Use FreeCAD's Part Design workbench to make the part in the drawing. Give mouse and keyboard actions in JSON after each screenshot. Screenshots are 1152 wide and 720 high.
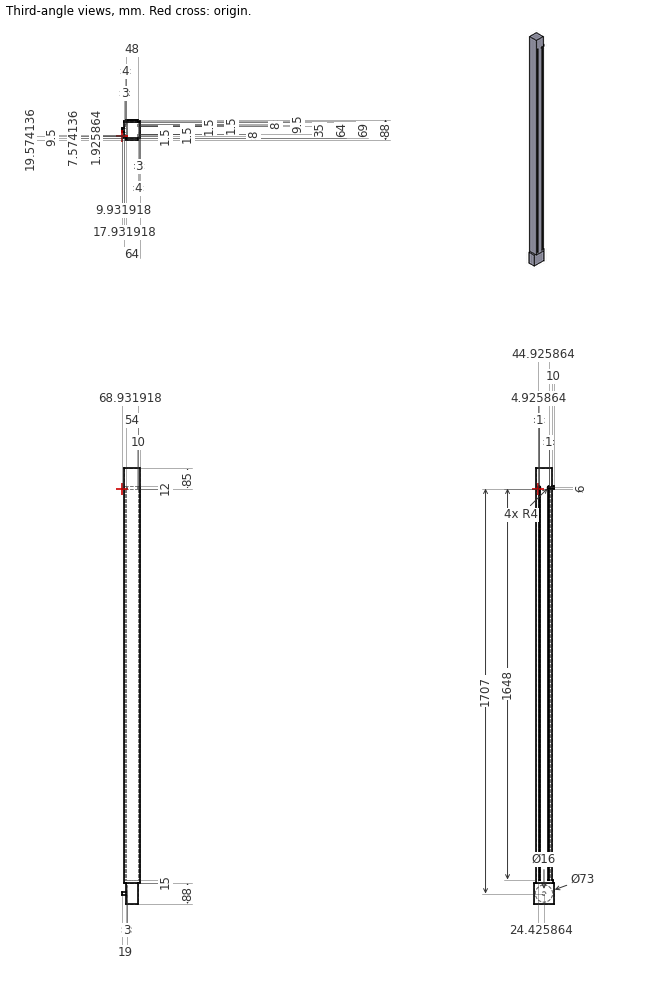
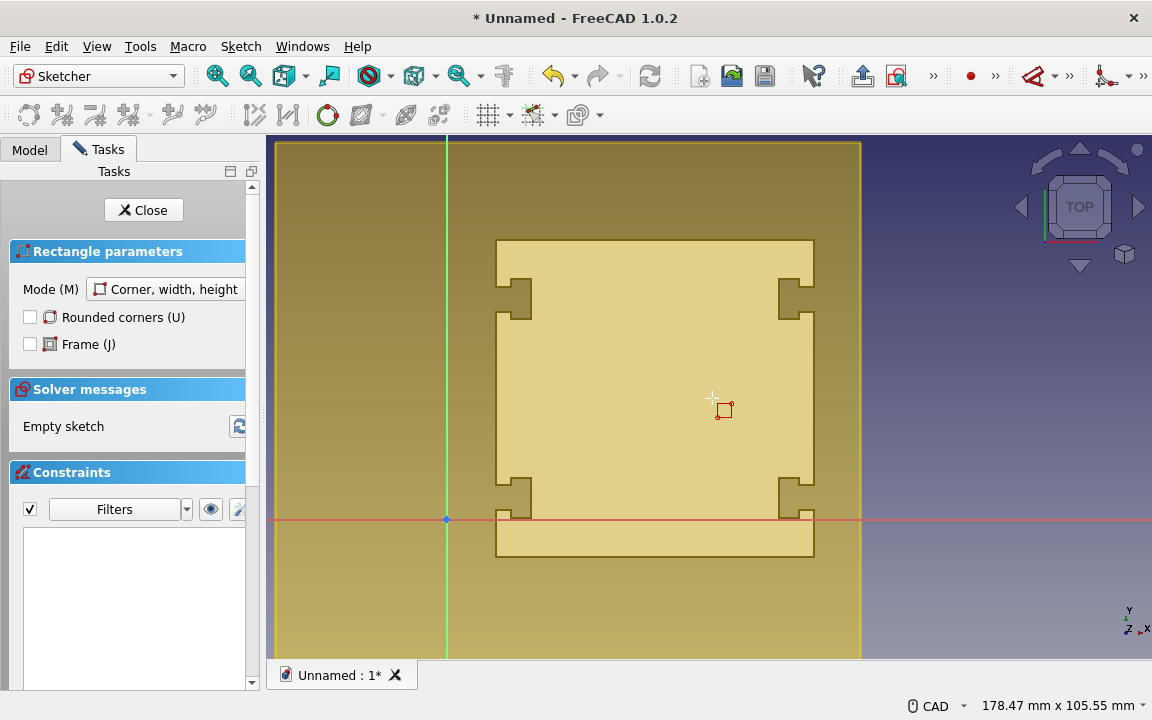
{"action": "left_click", "coordinate": [496, 215]}
{"action": "mouse_move", "coordinate": [814, 557]}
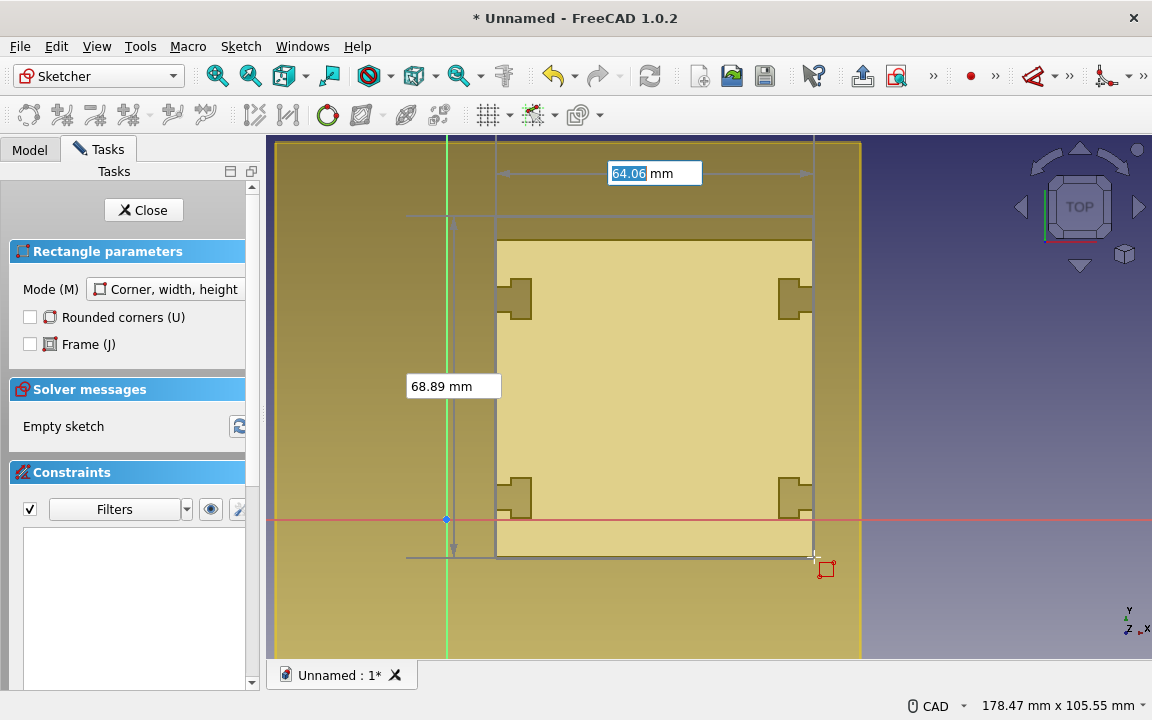
{"action": "type", "text": "64"}
{"action": "key", "text": "Tab"}
{"action": "type", "text": "69"}
{"action": "key", "text": "Return"}
{"action": "key", "text": "Escape"}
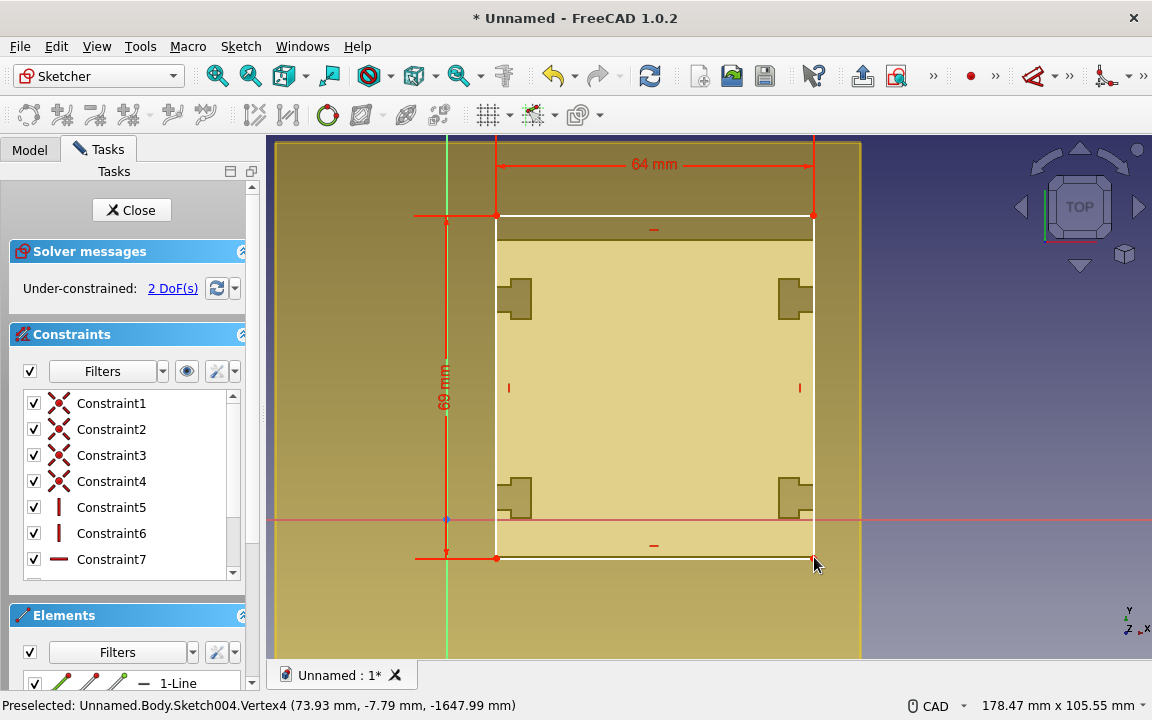
{"action": "left_click", "coordinate": [1032, 76]}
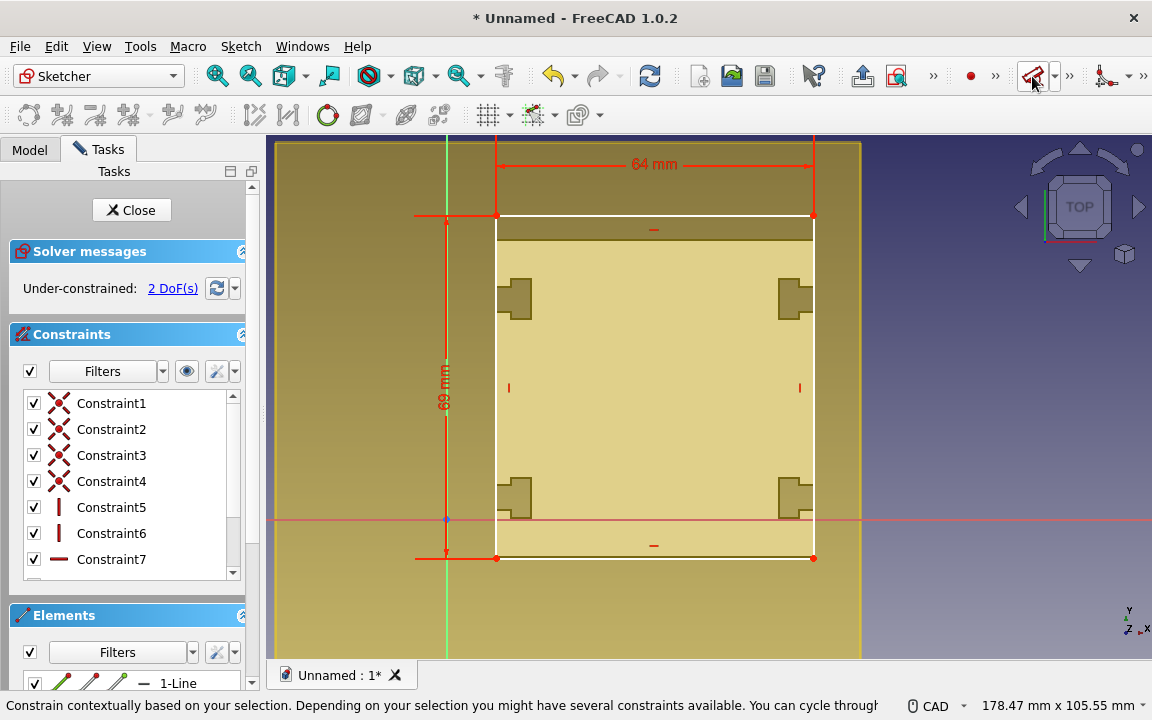
{"action": "left_click", "coordinate": [496, 216]}
{"action": "left_click", "coordinate": [471, 182]}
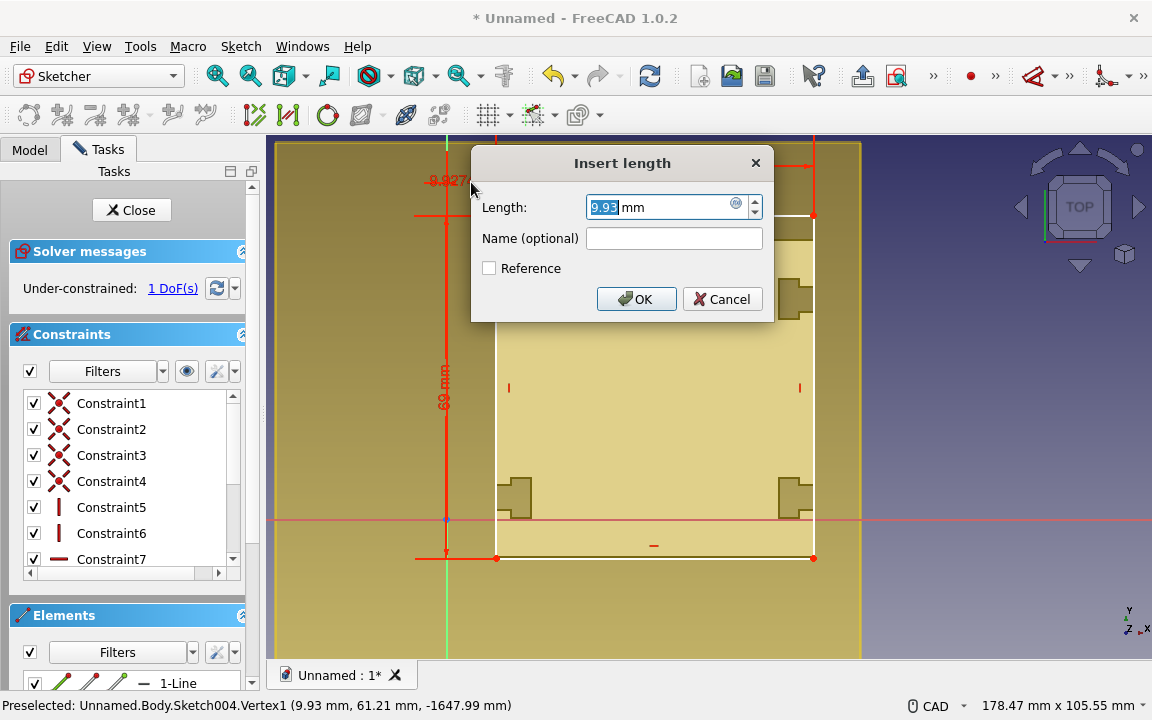
{"action": "type", "text": "9.931918"}
{"action": "key", "text": "Return"}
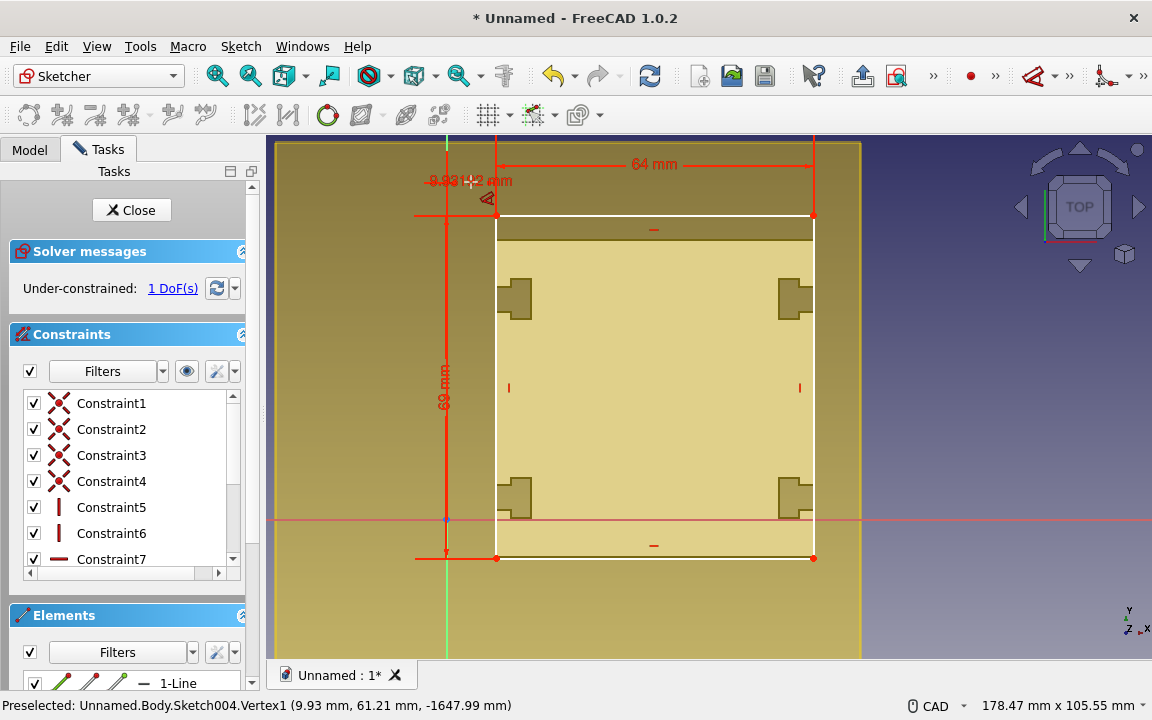
{"action": "left_click", "coordinate": [496, 559]}
{"action": "left_click", "coordinate": [413, 539]}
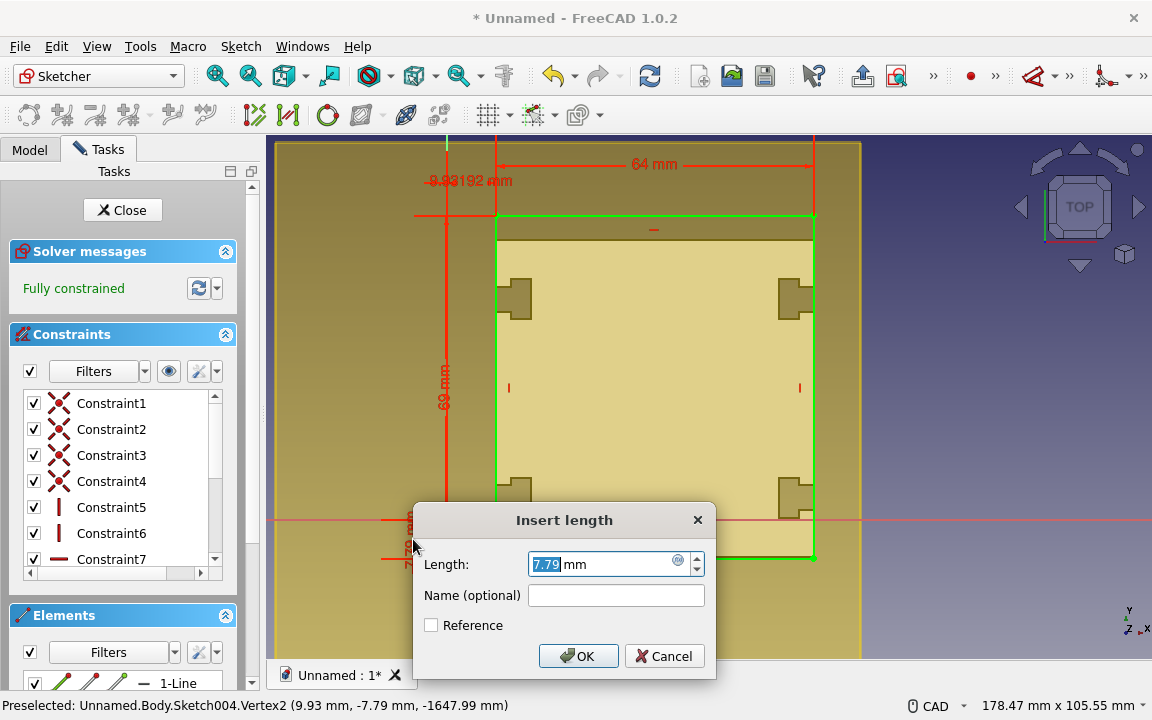
{"action": "type", "text": "7.574136"}
{"action": "key", "text": "Return"}
{"action": "key", "text": "Escape"}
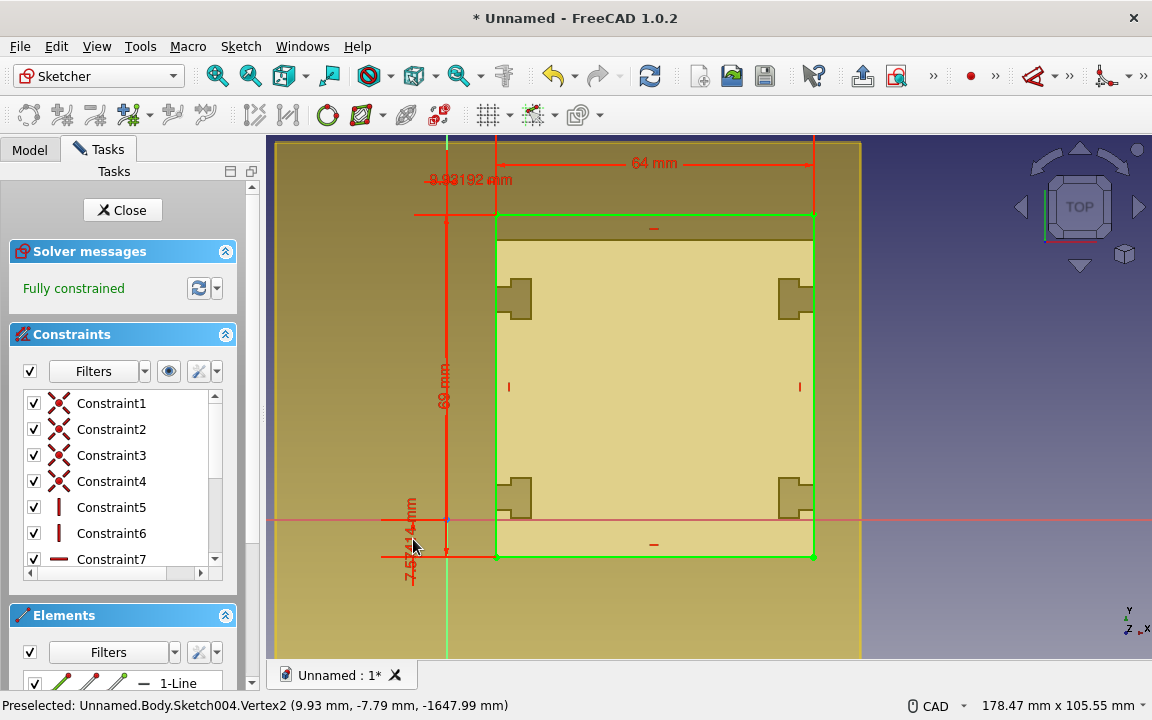
{"action": "left_click", "coordinate": [123, 210]}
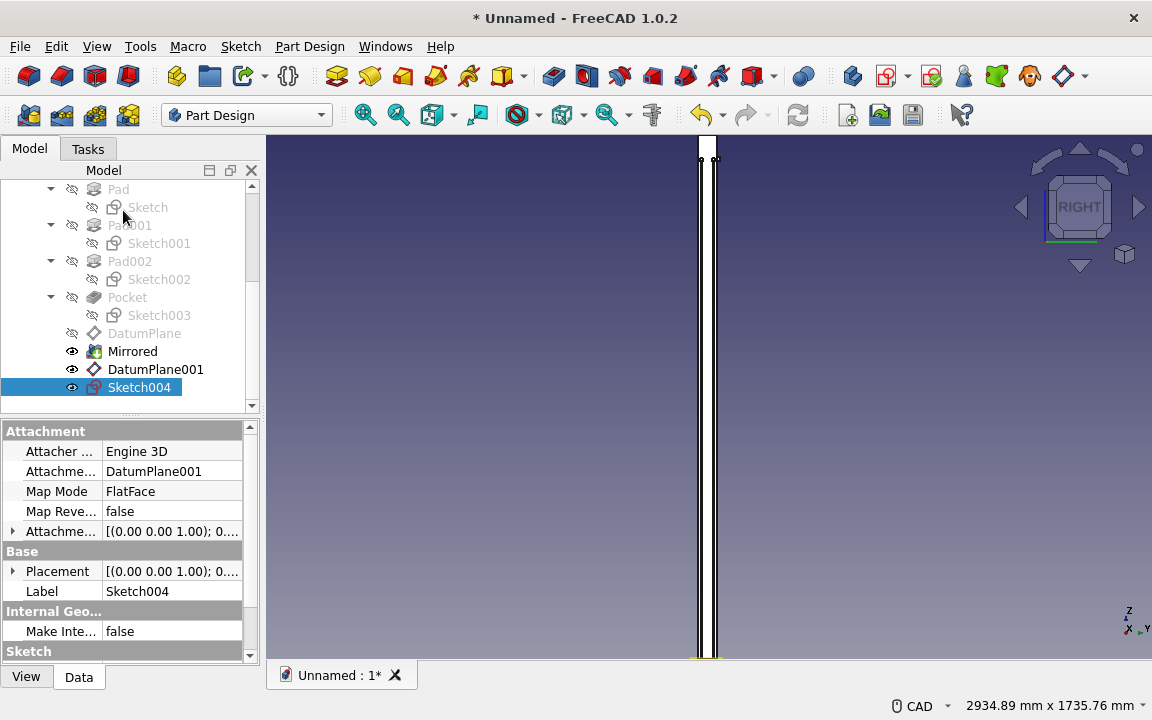
{"action": "left_click", "coordinate": [337, 76]}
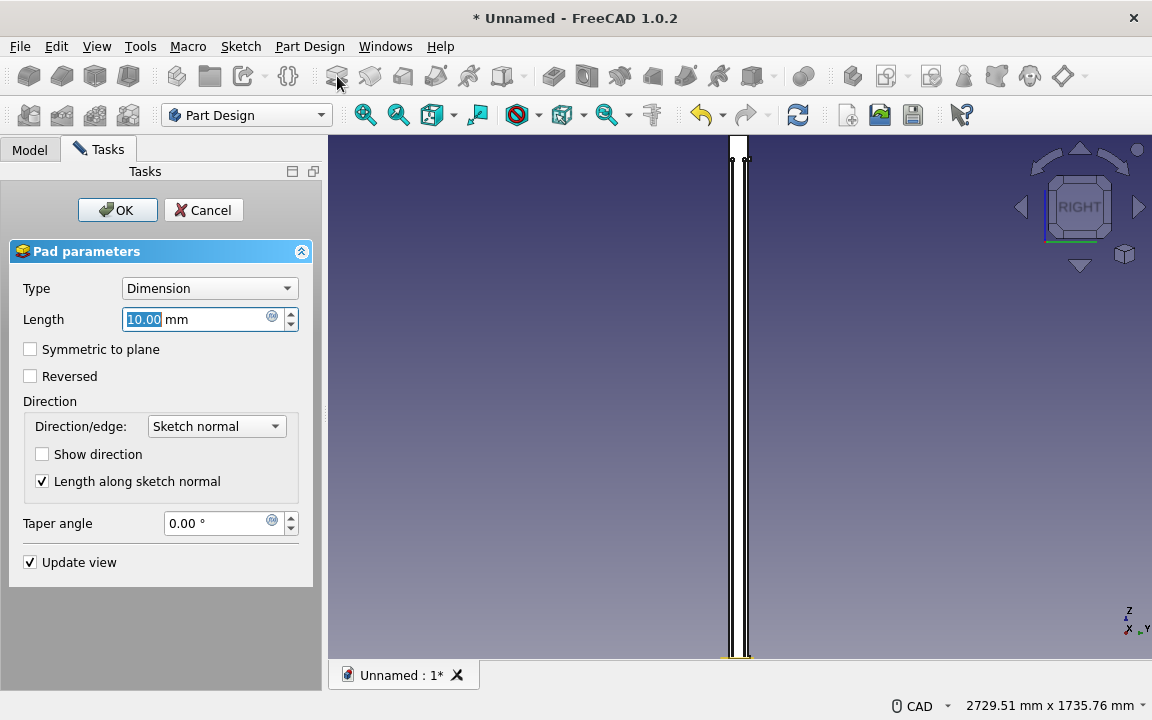
{"action": "type", "text": "15"}
{"action": "key", "text": "Tab"}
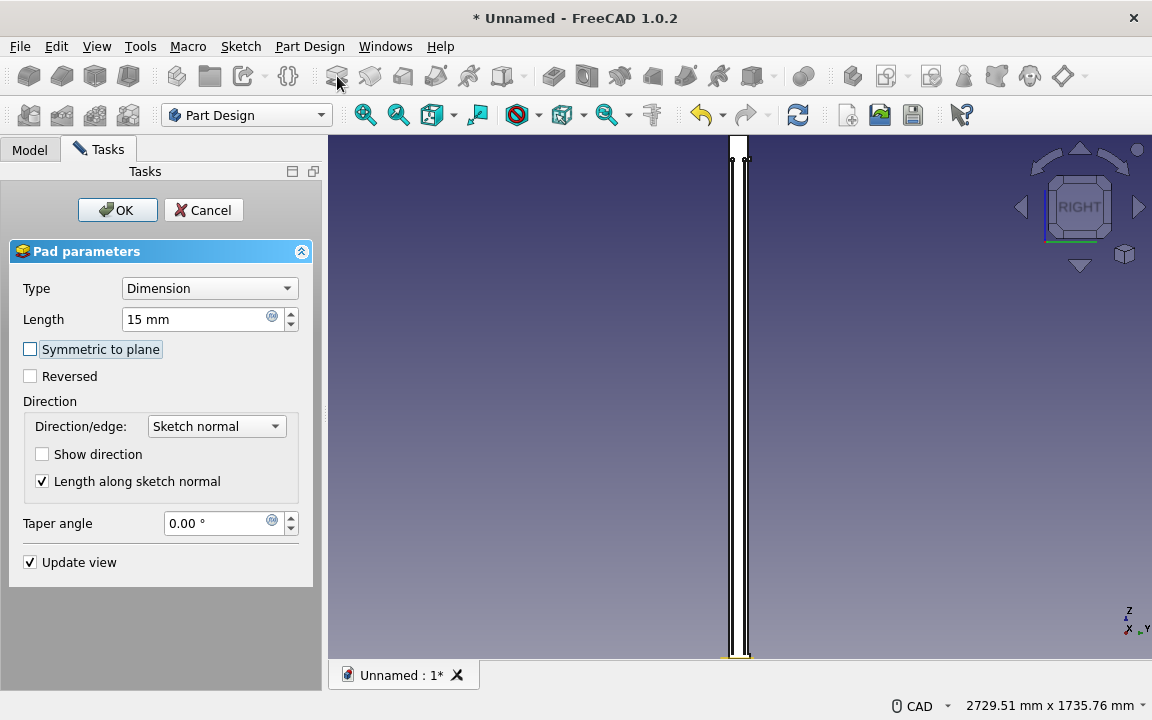
{"action": "left_click", "coordinate": [31, 376]}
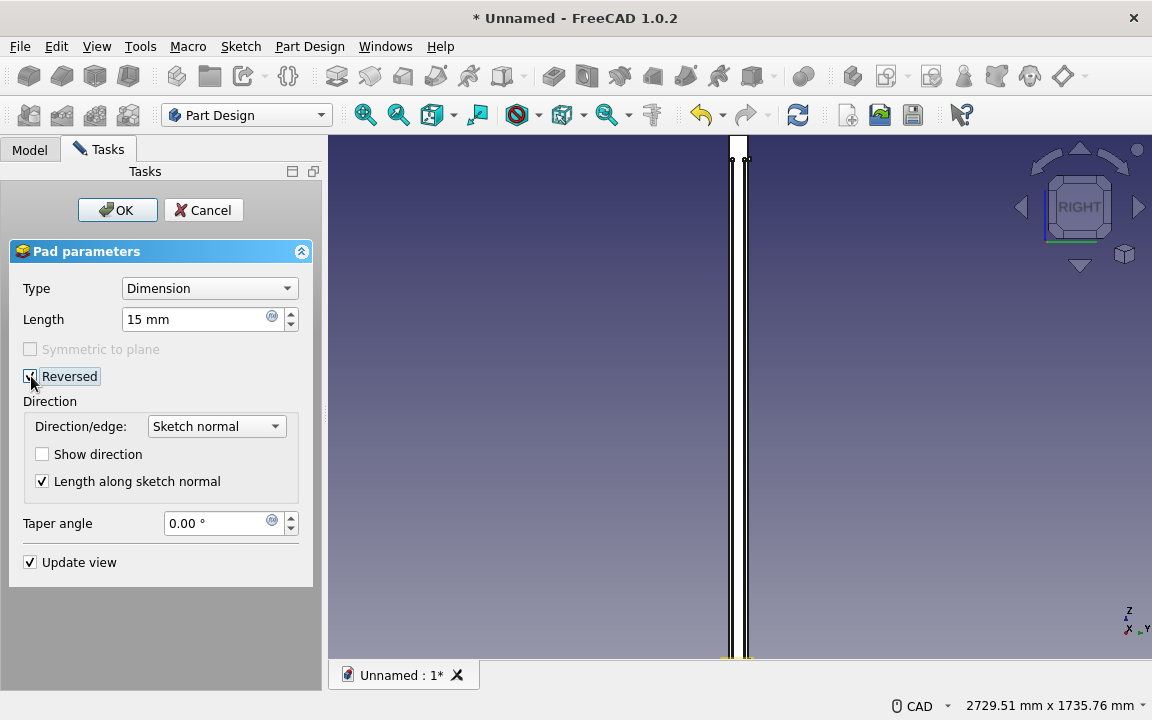
{"action": "left_click", "coordinate": [118, 210]}